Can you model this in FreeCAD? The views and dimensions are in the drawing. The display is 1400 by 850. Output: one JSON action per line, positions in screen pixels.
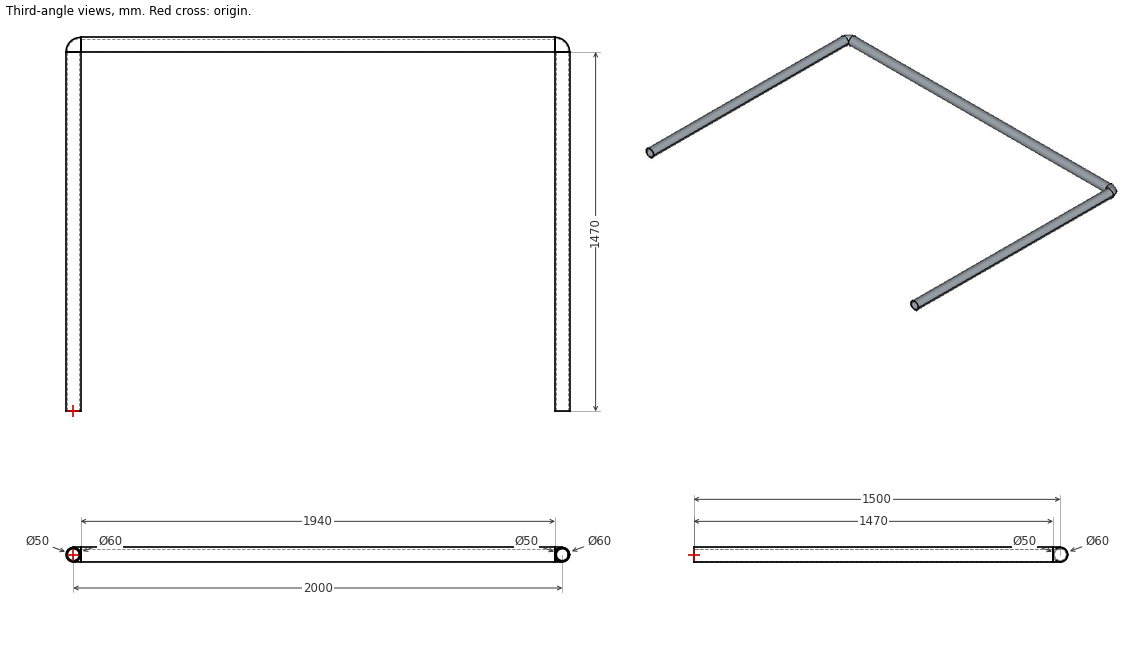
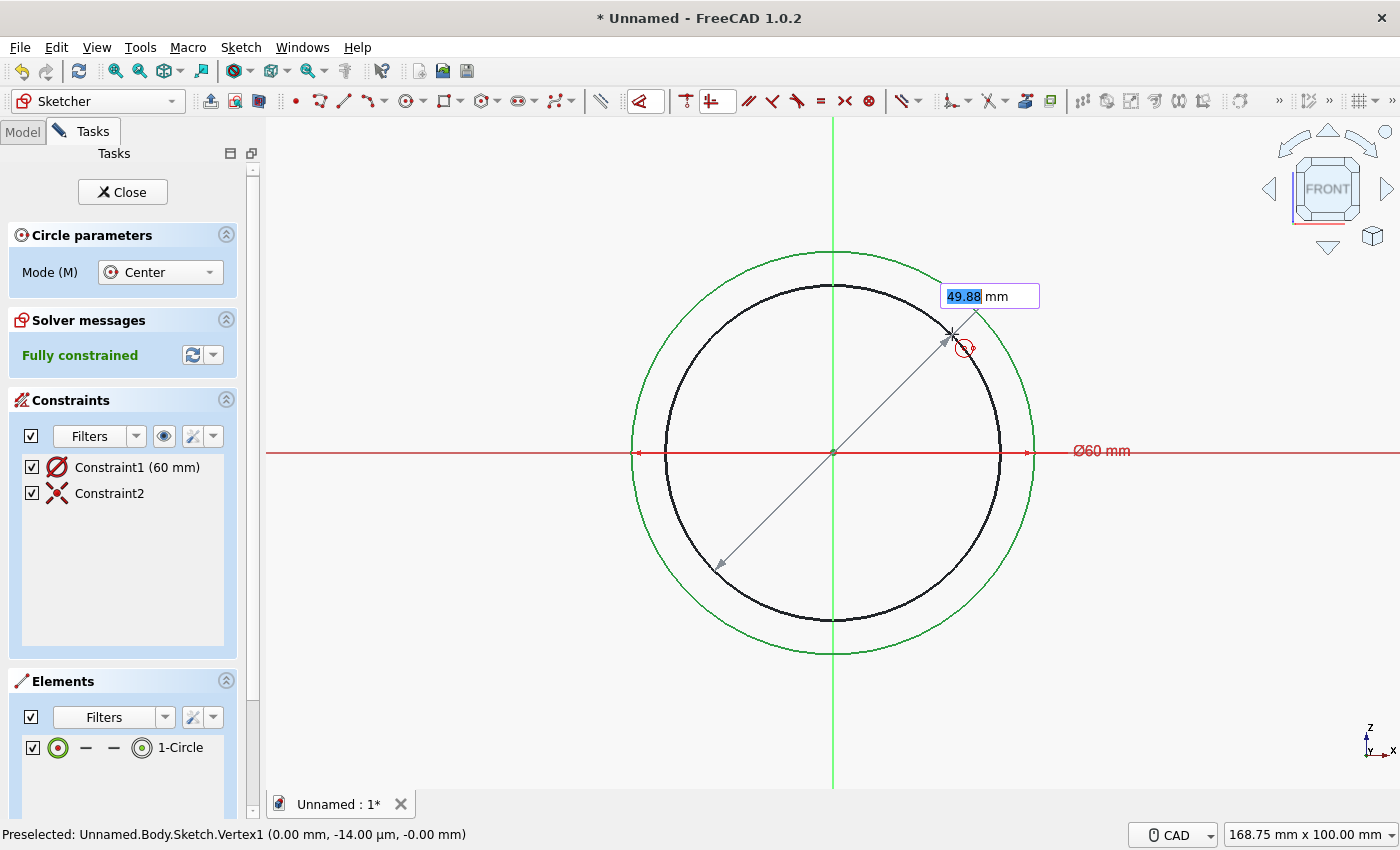
{"action": "type", "text": "50"}
{"action": "key", "text": "Return"}
{"action": "key", "text": "Escape"}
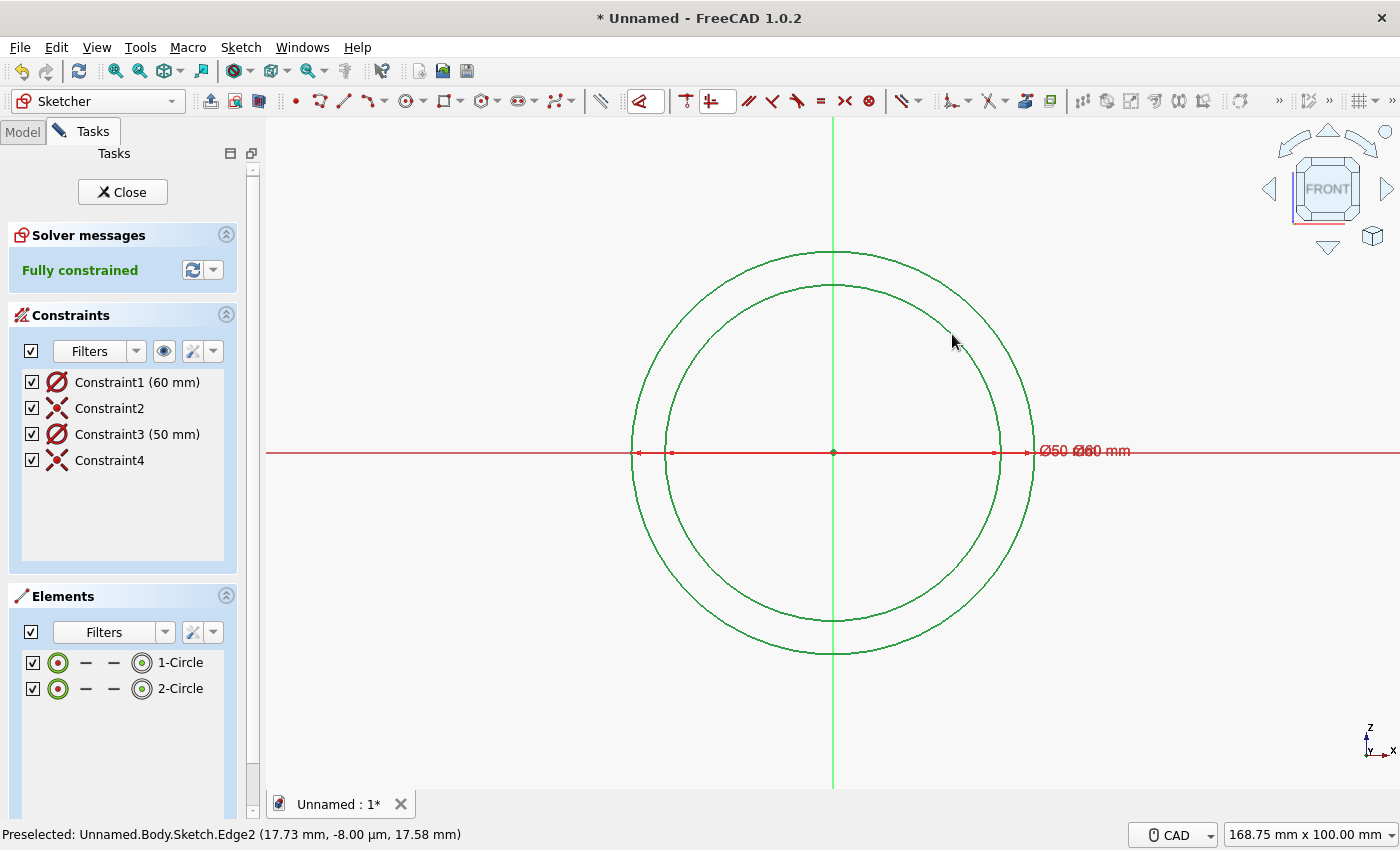
{"action": "left_click", "coordinate": [123, 192]}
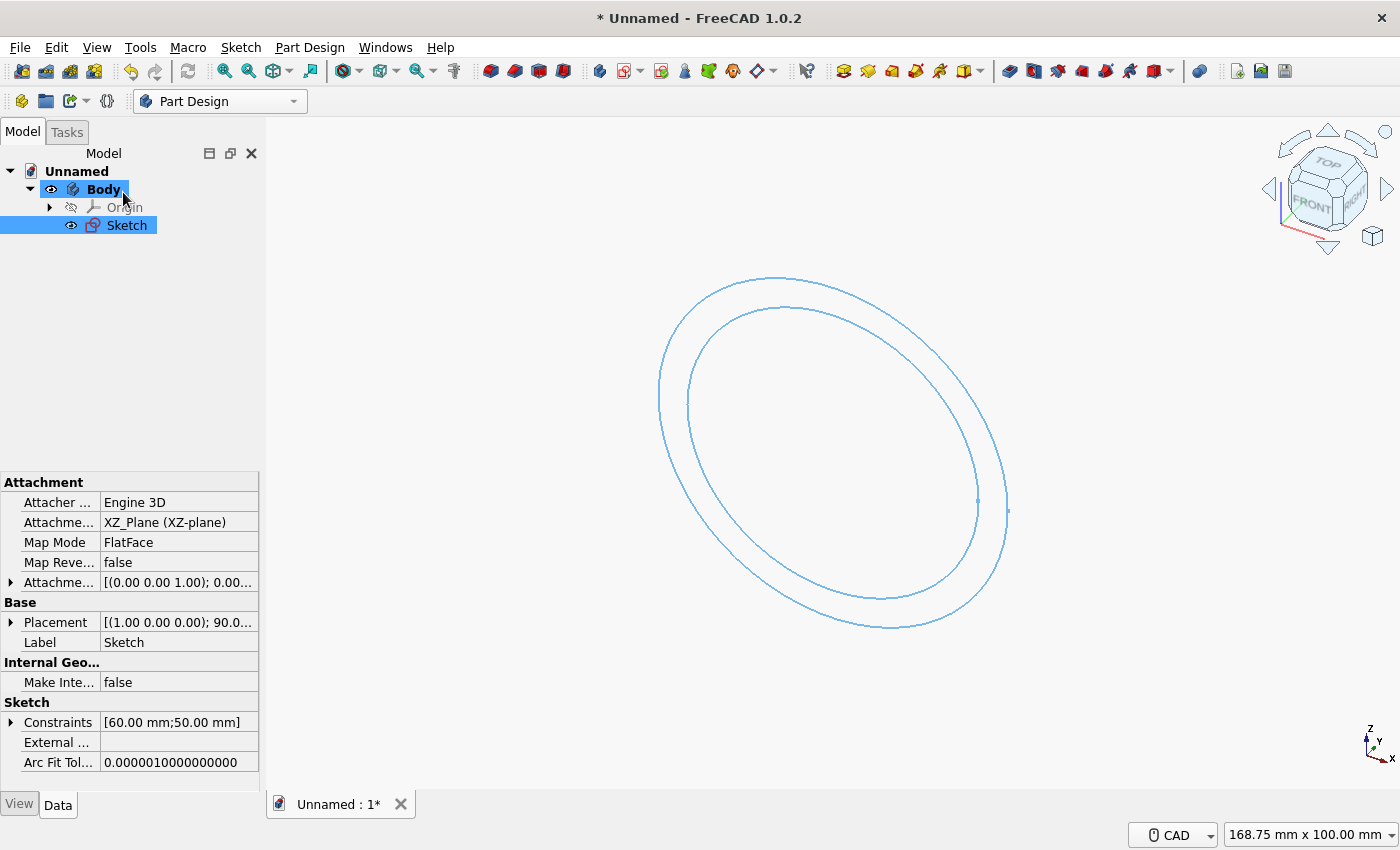
{"action": "left_click", "coordinate": [844, 72]}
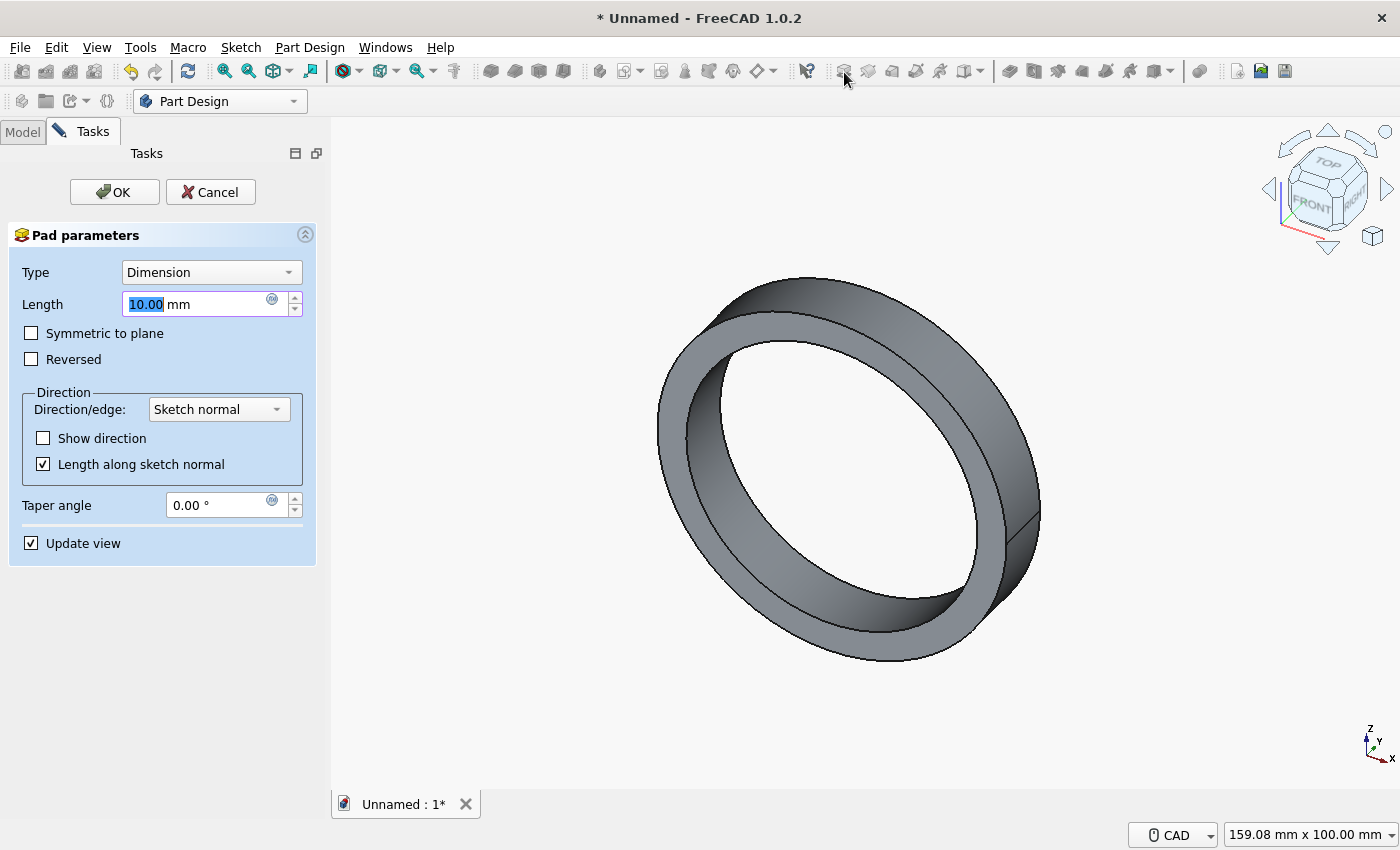
{"action": "type", "text": "1470"}
{"action": "key", "text": "Tab"}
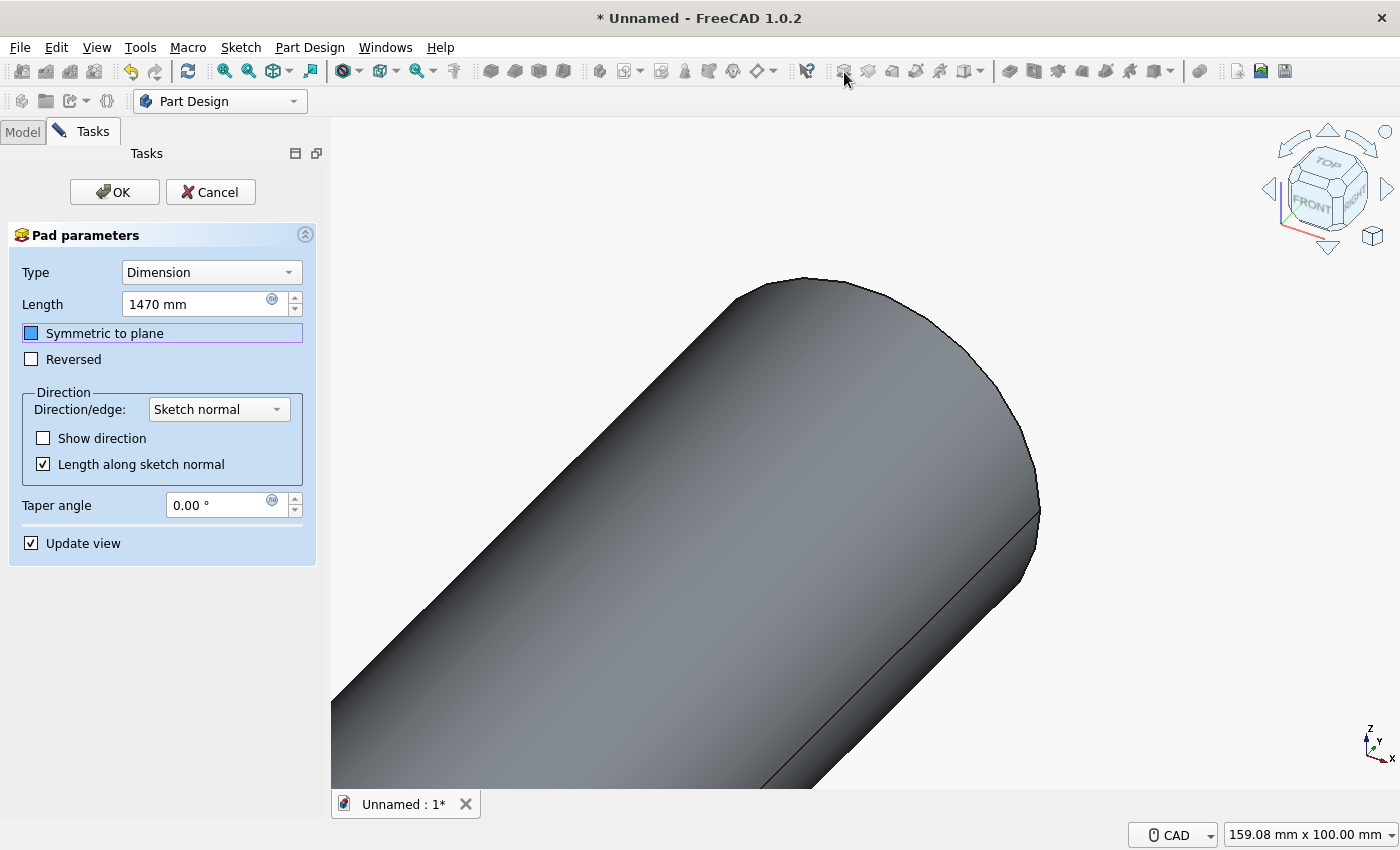
{"action": "left_click", "coordinate": [30, 359]}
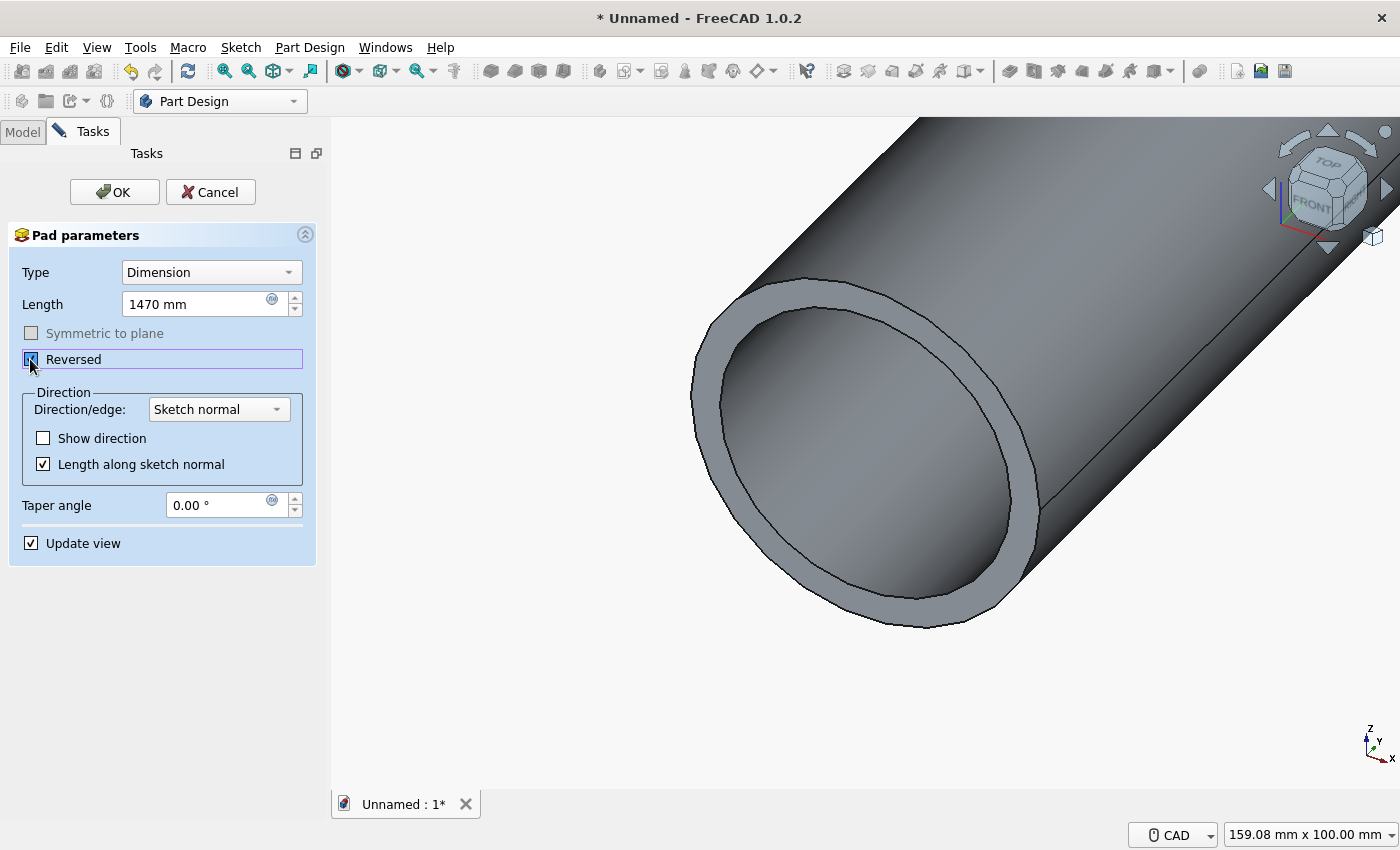
{"action": "left_click", "coordinate": [115, 192]}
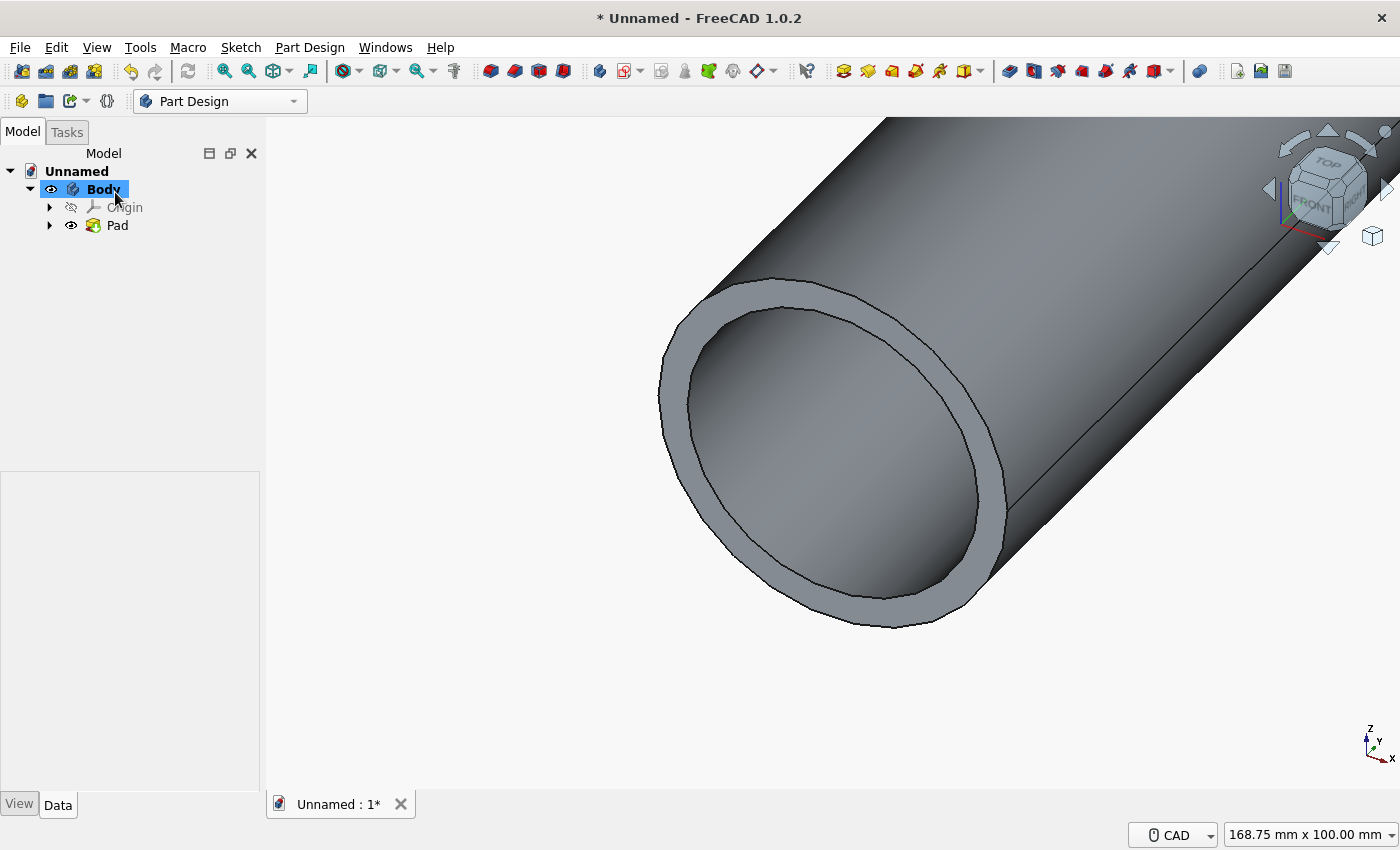
{"action": "key", "text": "v f"}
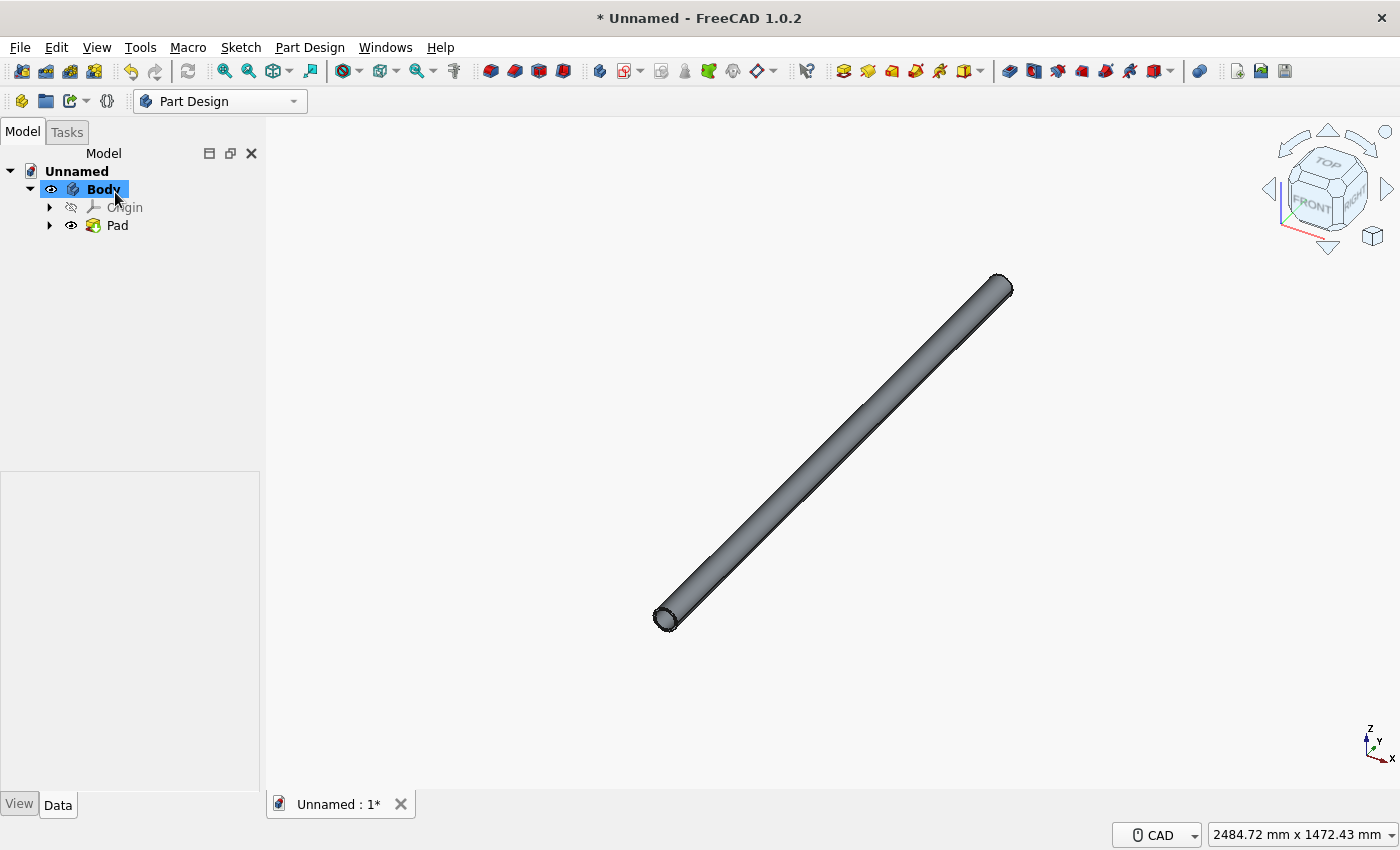
{"action": "left_click", "coordinate": [600, 72]}